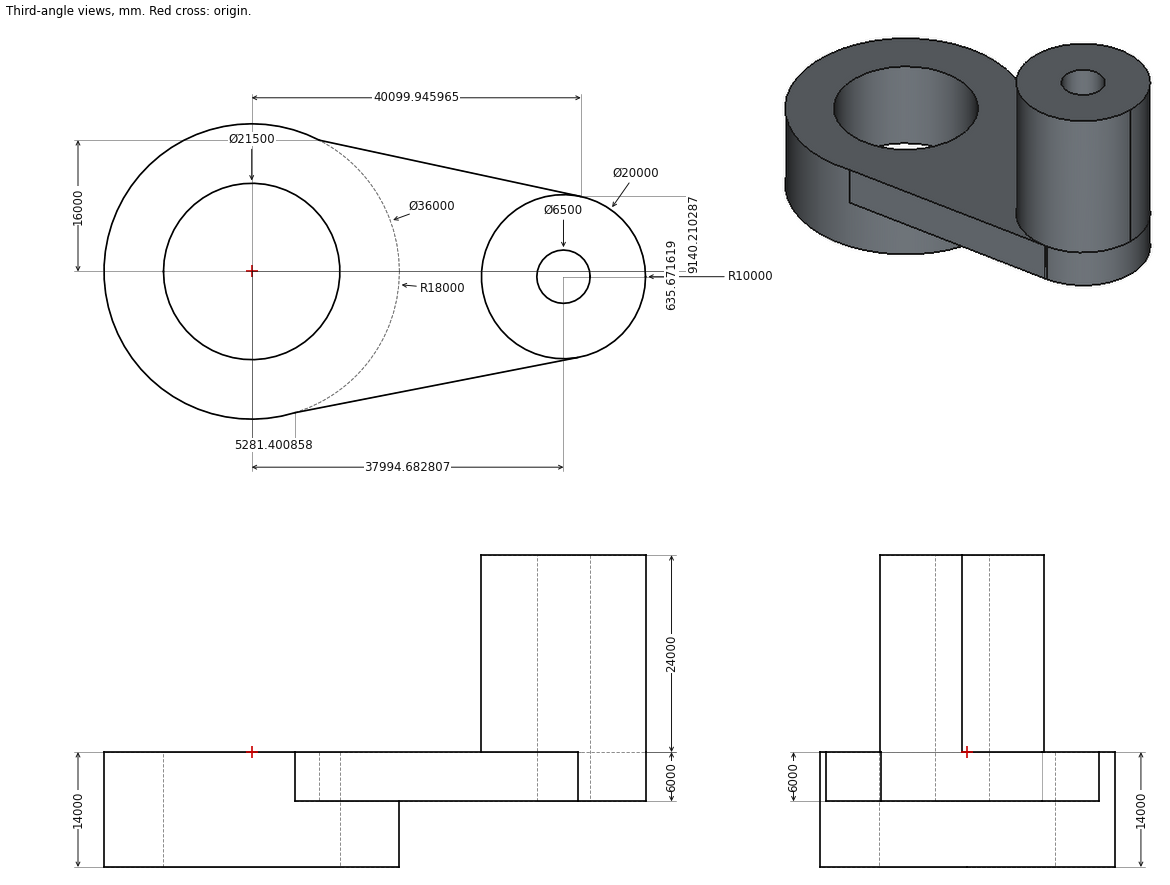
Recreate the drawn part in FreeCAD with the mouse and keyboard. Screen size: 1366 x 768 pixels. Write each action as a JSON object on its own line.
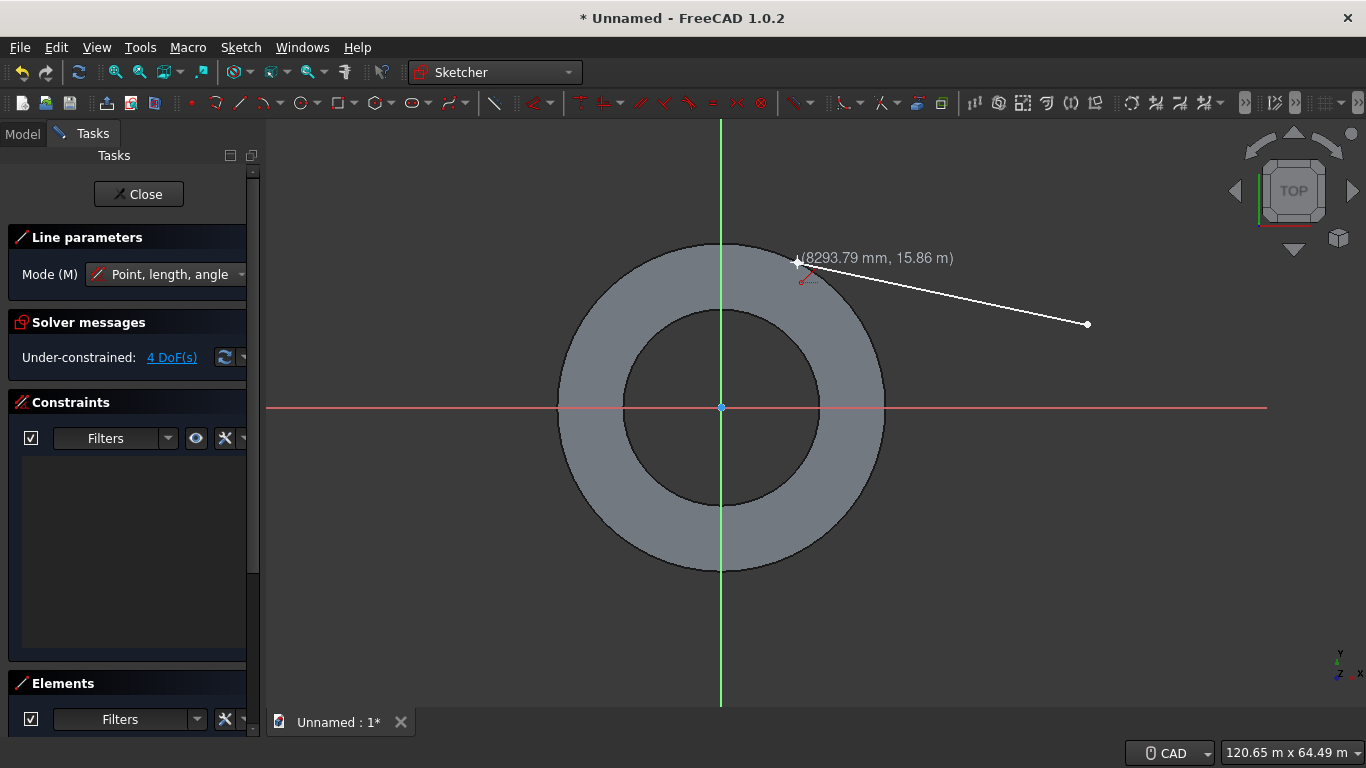
{"action": "left_click", "coordinate": [770, 565]}
{"action": "left_click", "coordinate": [1087, 503]}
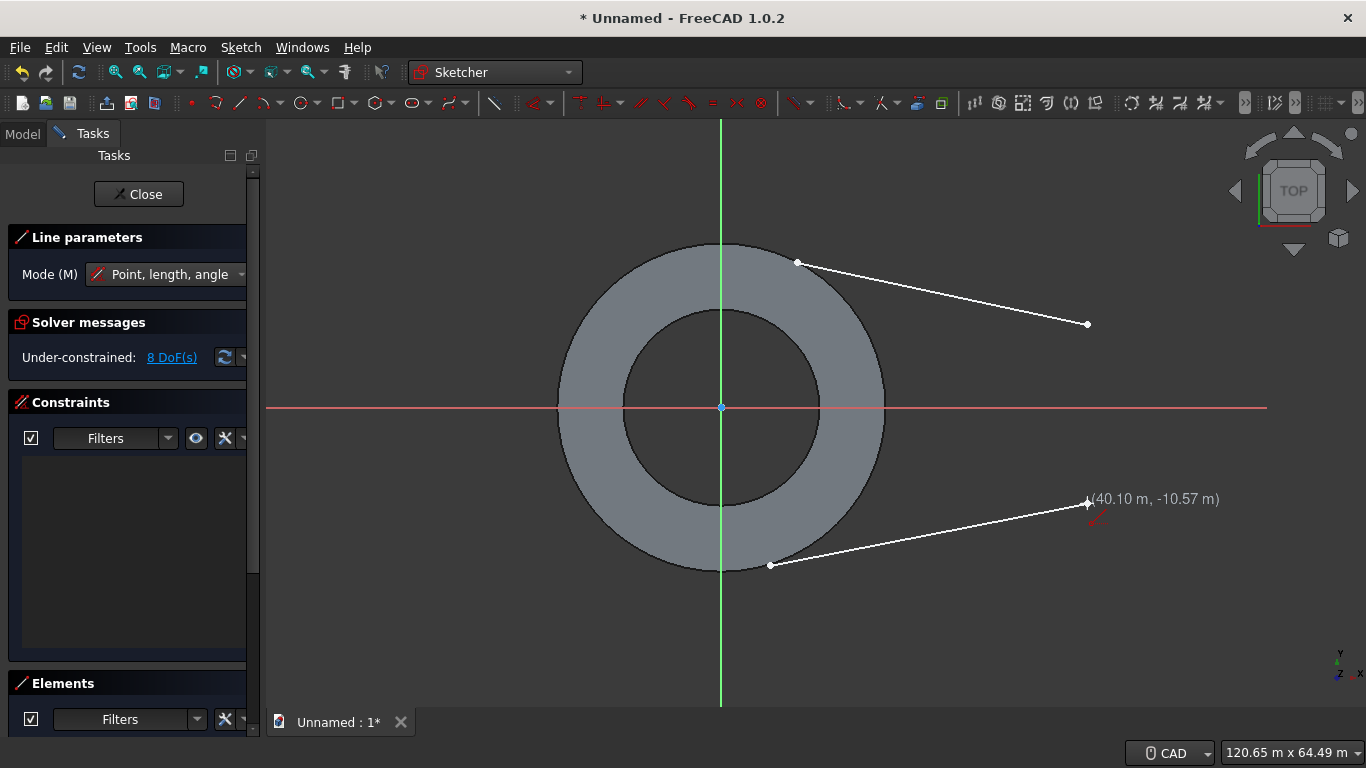
{"action": "key", "text": "g 3 a"}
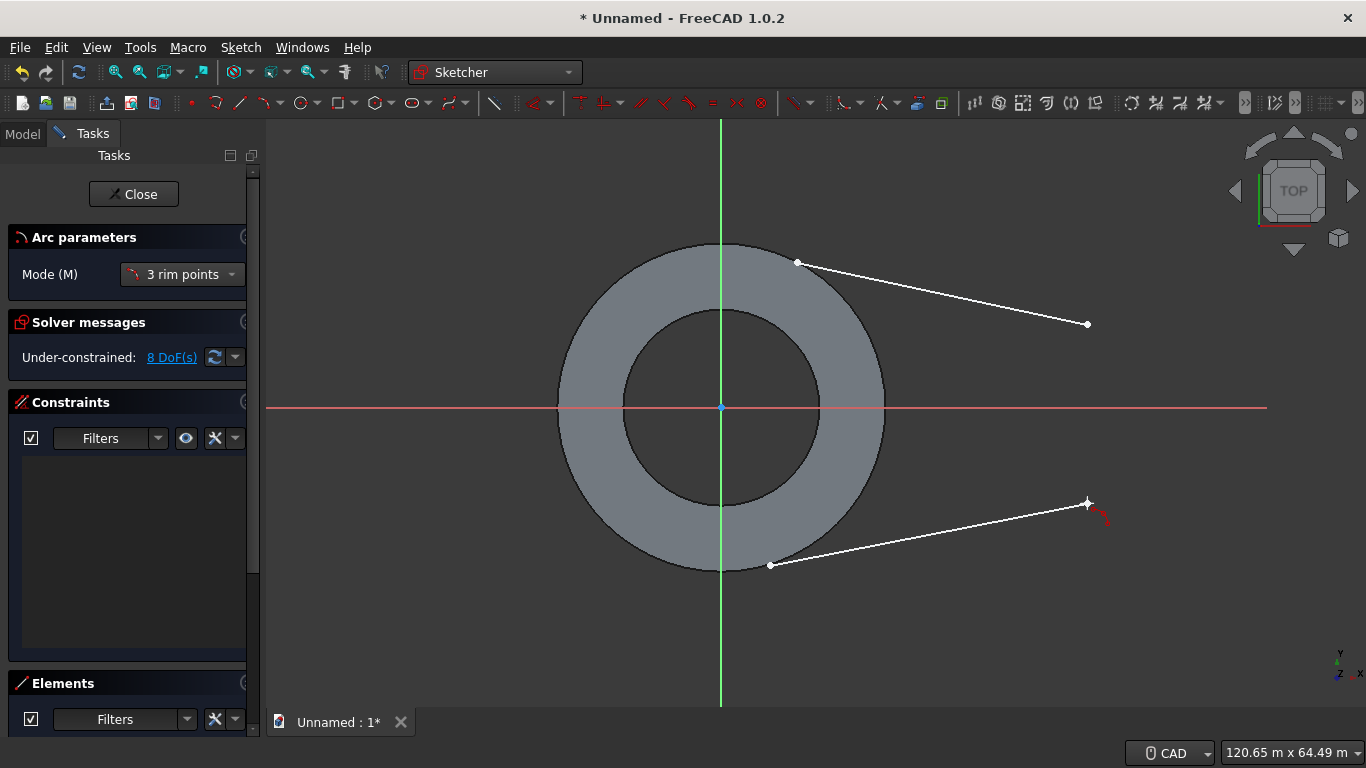
{"action": "left_click", "coordinate": [797, 263]}
{"action": "left_click", "coordinate": [770, 566]}
{"action": "left_click", "coordinate": [885, 422]}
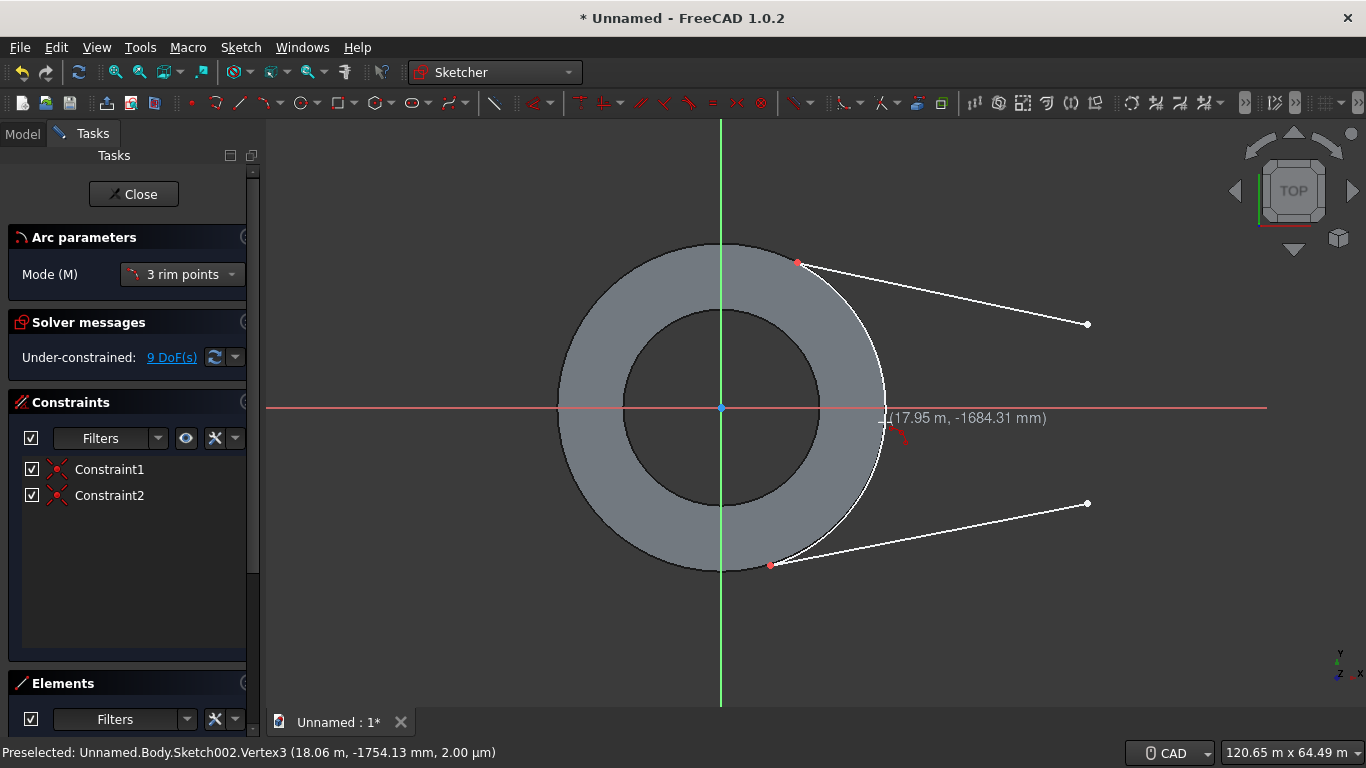
{"action": "left_click", "coordinate": [1087, 504]}
{"action": "left_click", "coordinate": [1087, 325]}
{"action": "left_click", "coordinate": [1156, 438]}
{"action": "key", "text": "Escape"}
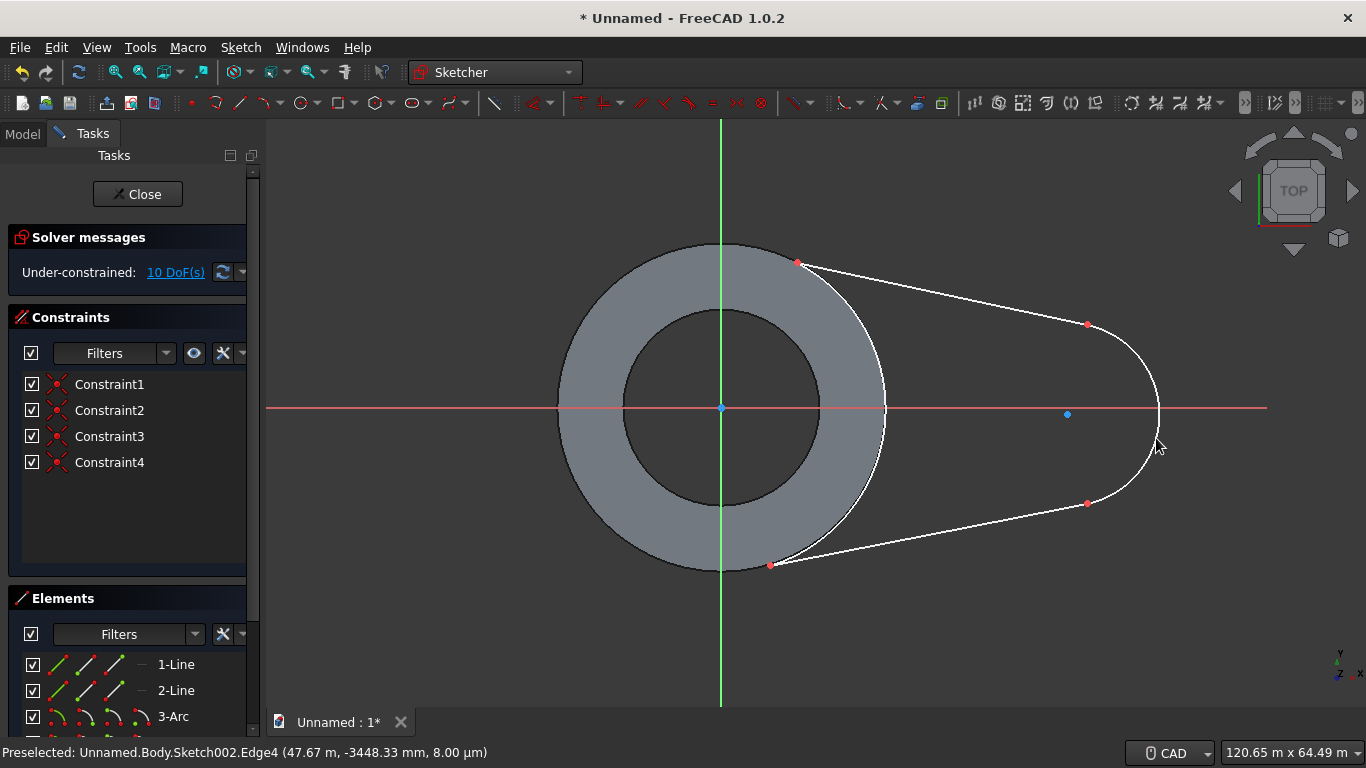
{"action": "left_click_drag", "start_coordinate": [711, 398], "coordinate": [731, 419]}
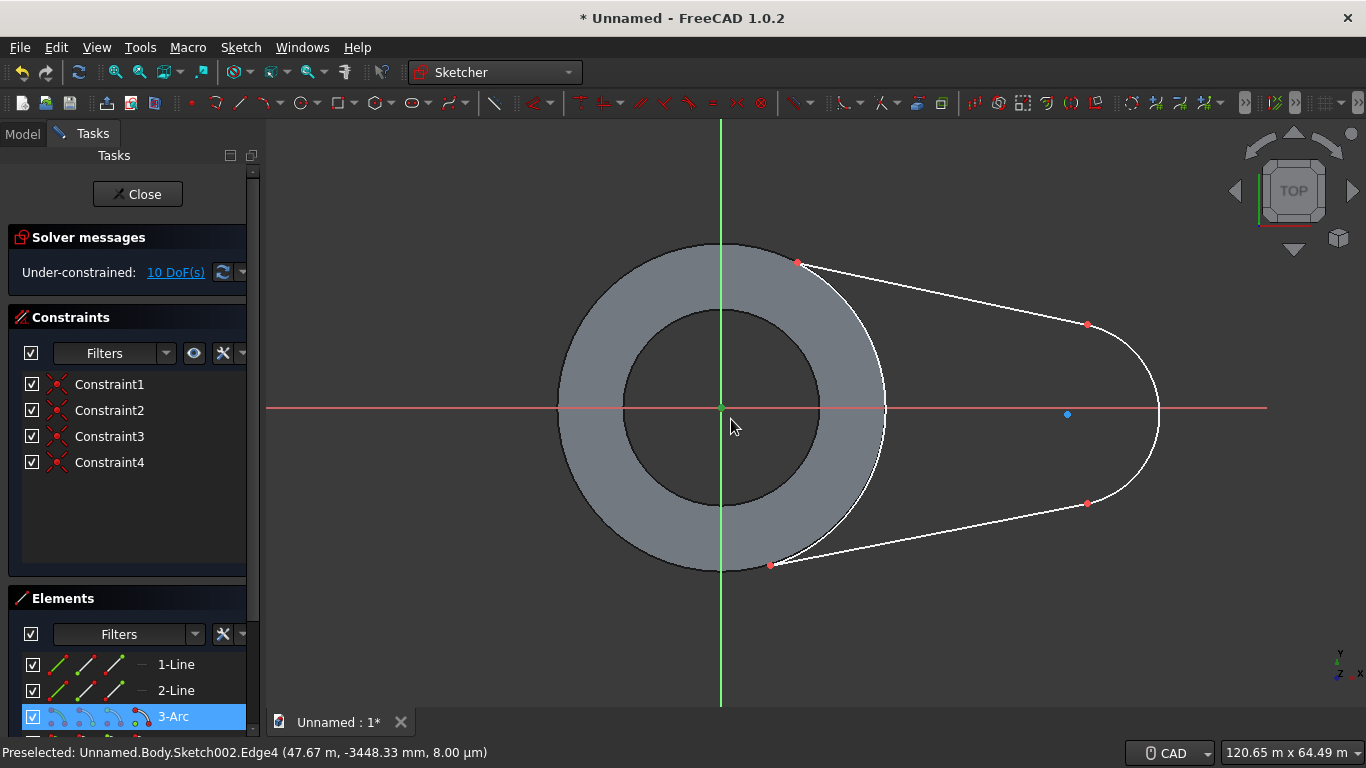
{"action": "left_click", "coordinate": [580, 104]}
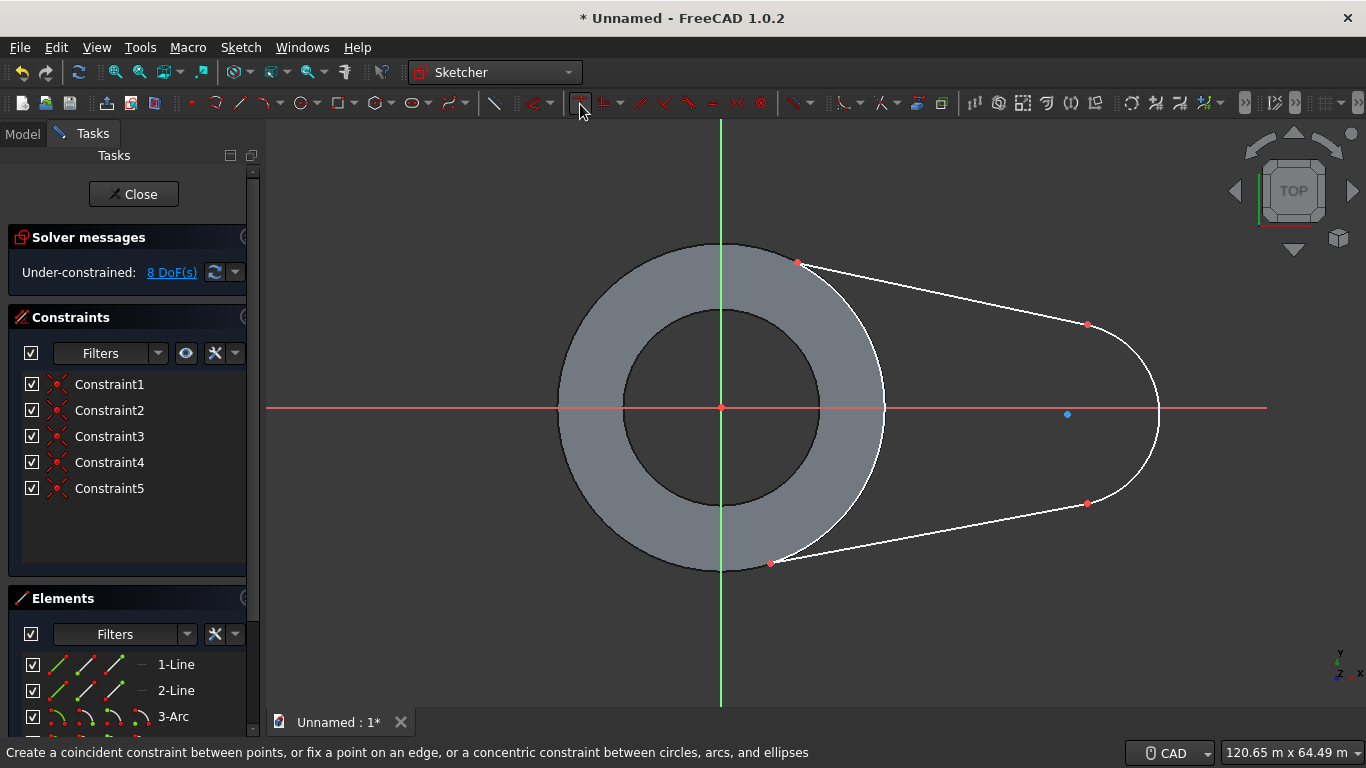
{"action": "left_click", "coordinate": [534, 104]}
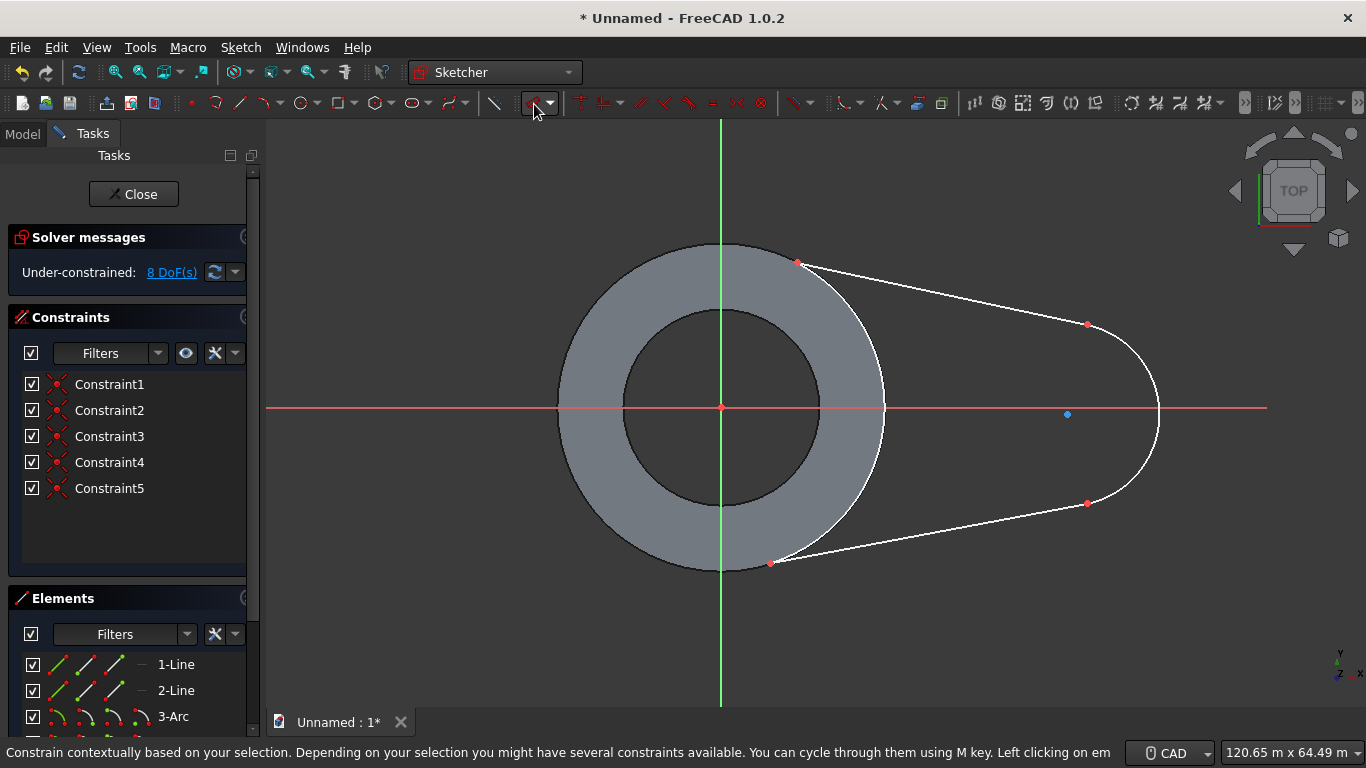
{"action": "left_click", "coordinate": [860, 494]}
{"action": "left_click", "coordinate": [887, 511]}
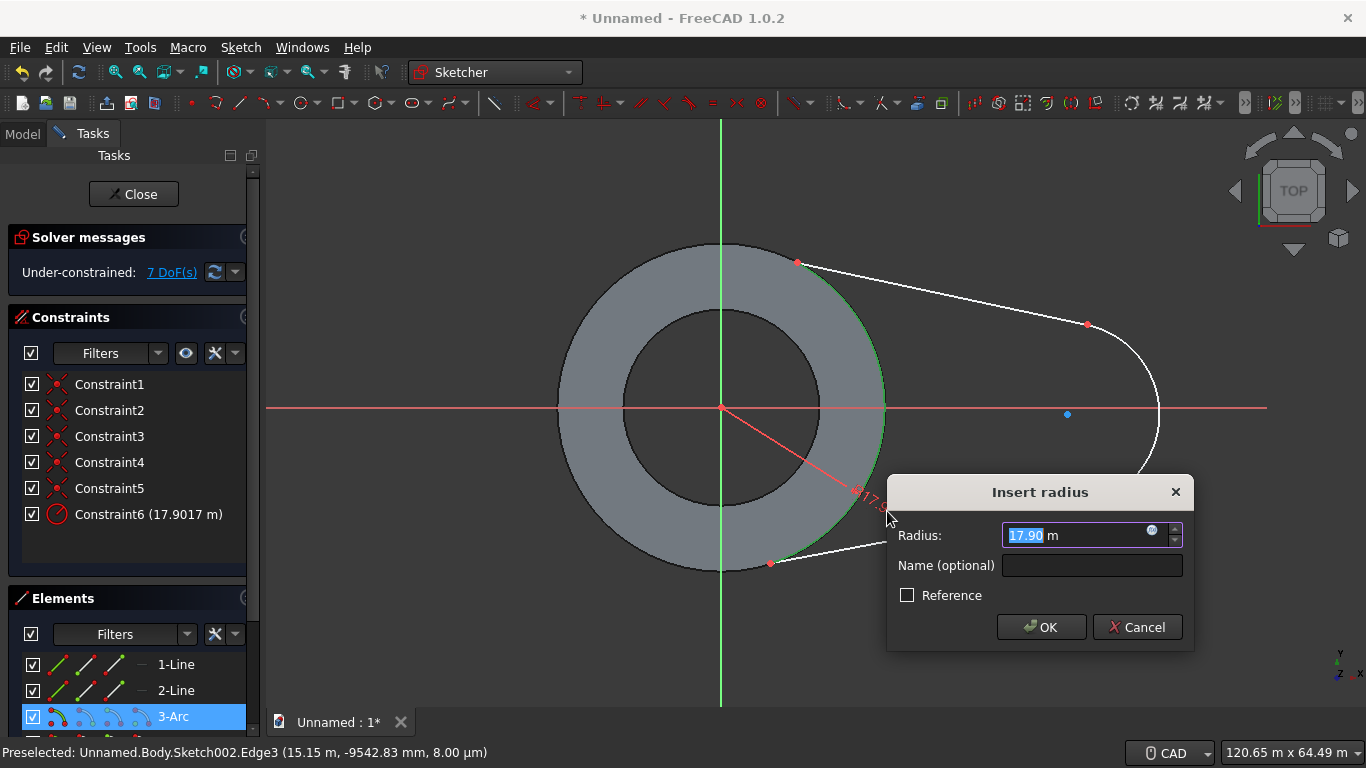
{"action": "key", "text": "ctrl+a"}
{"action": "type", "text": "18000 mm"}
{"action": "key", "text": "Return"}